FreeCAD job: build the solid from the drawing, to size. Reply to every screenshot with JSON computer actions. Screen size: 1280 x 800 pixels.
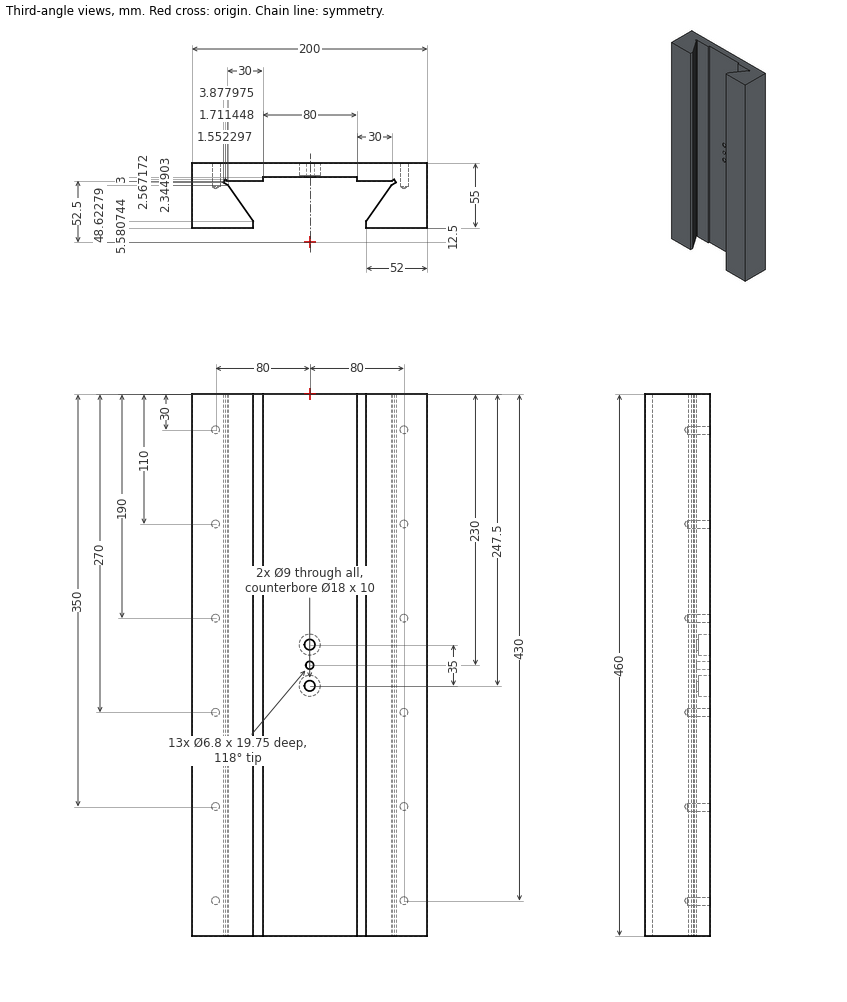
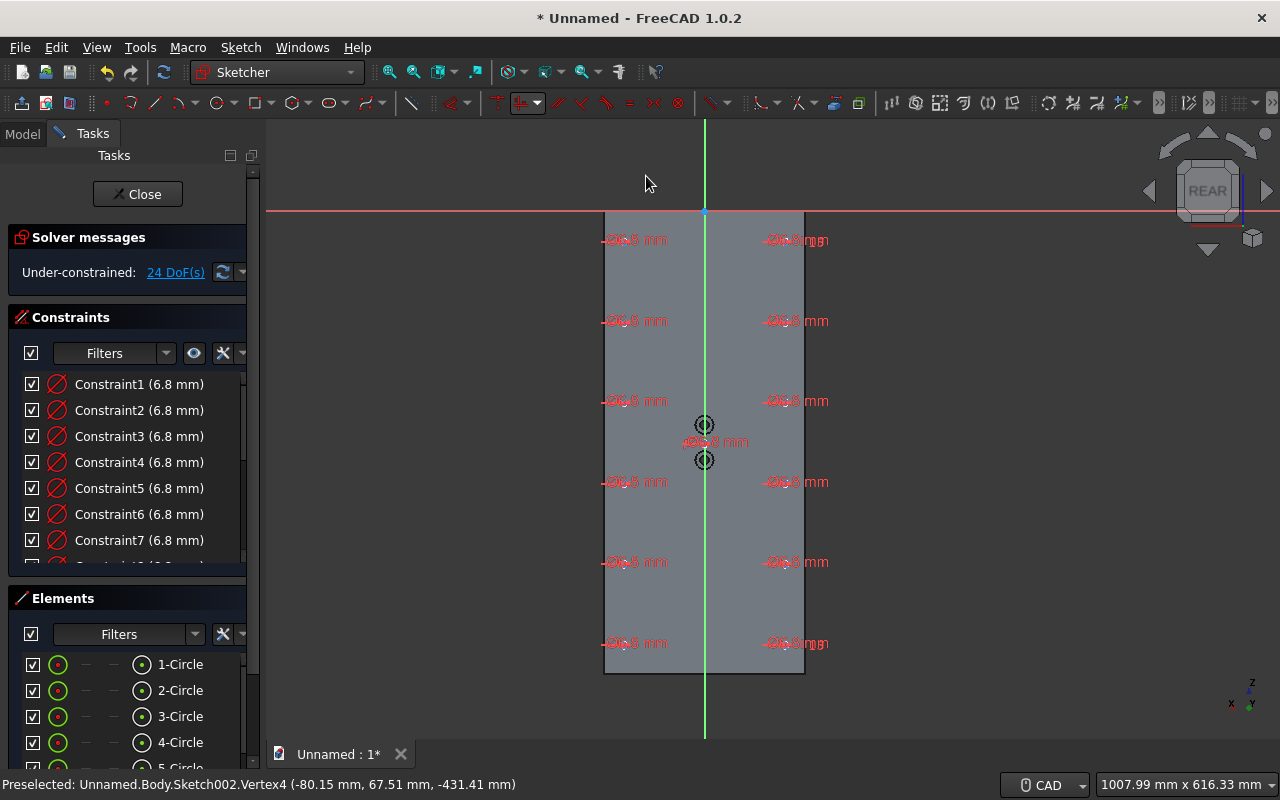
{"action": "left_click", "coordinate": [624, 645]}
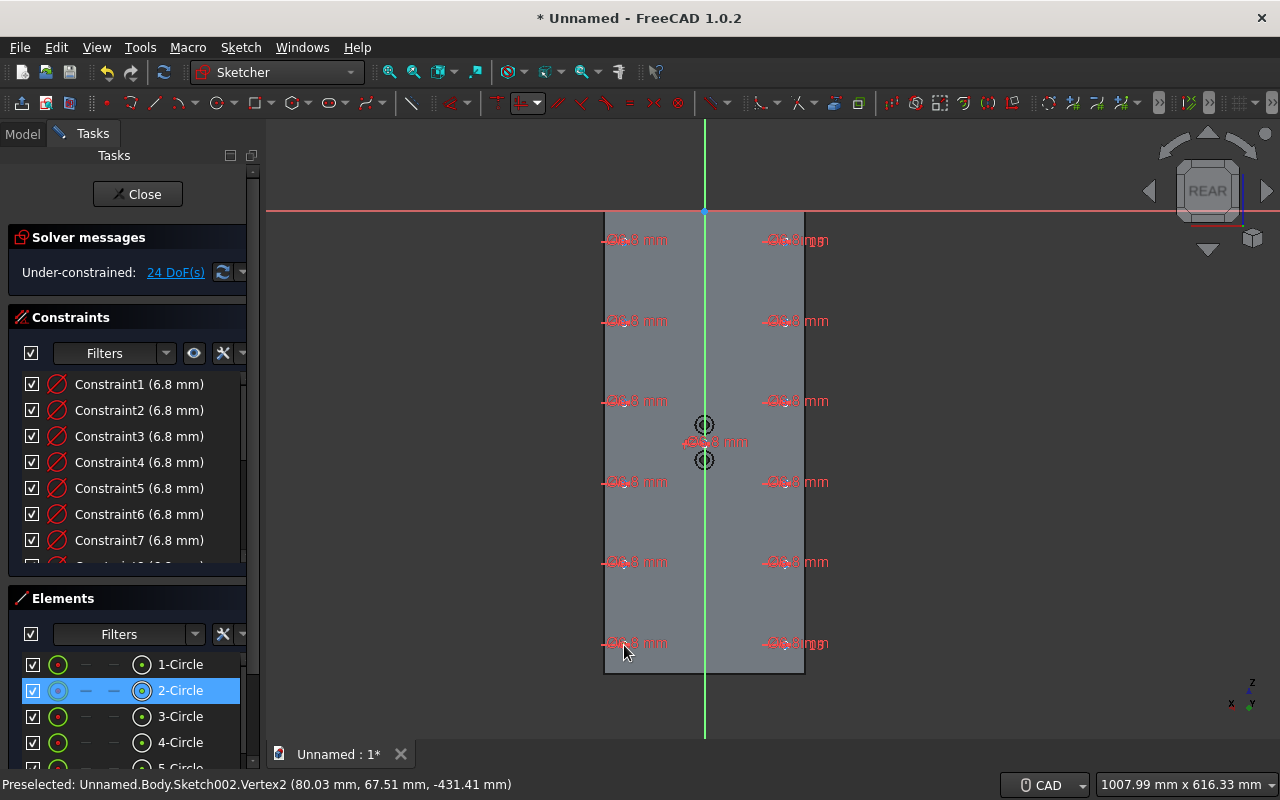
{"action": "left_click", "coordinate": [785, 645]}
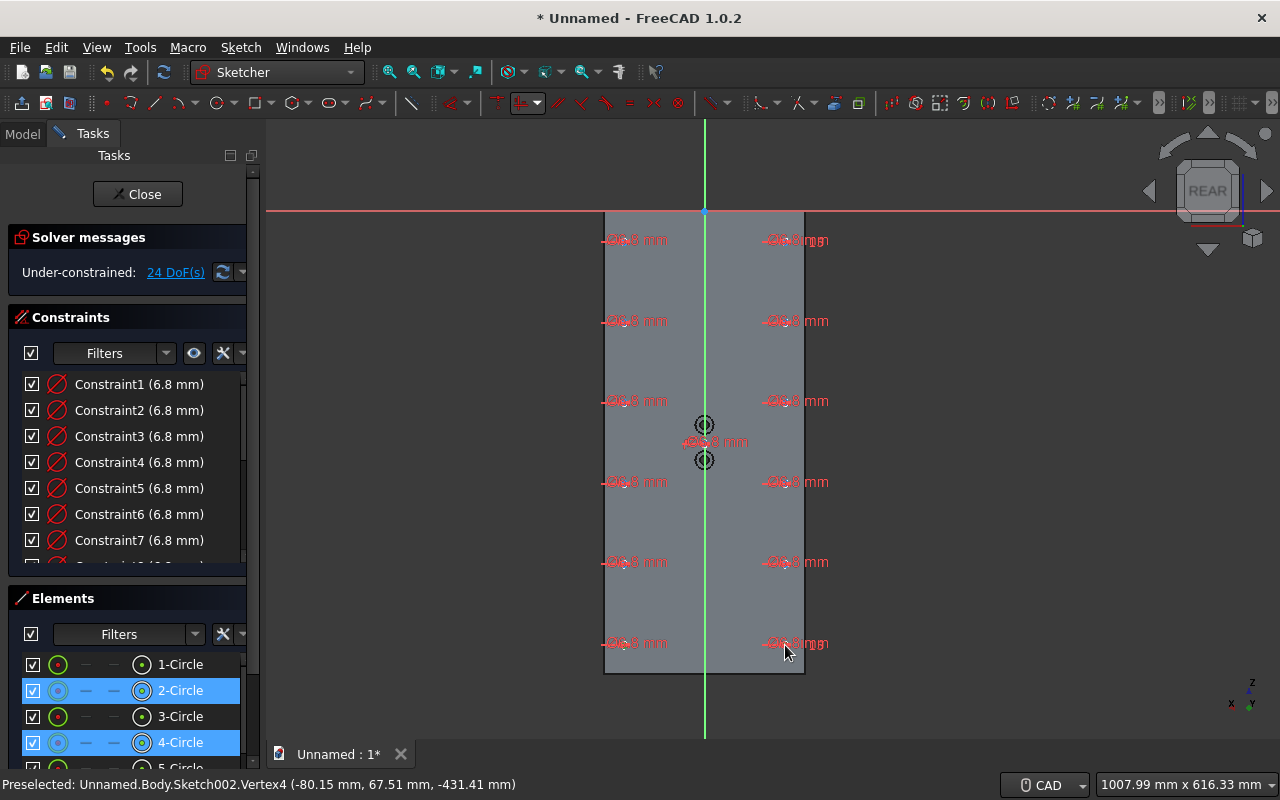
{"action": "key", "text": "h"}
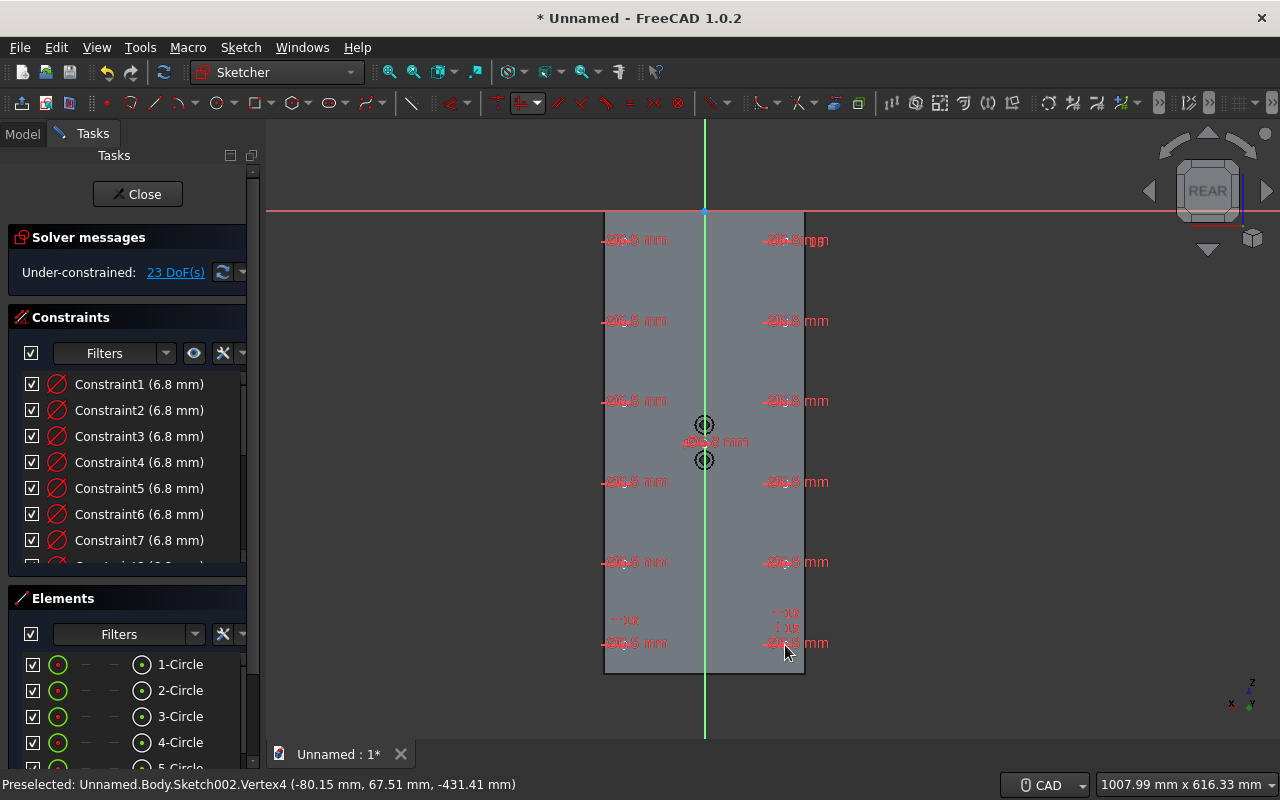
{"action": "left_click", "coordinate": [624, 645]}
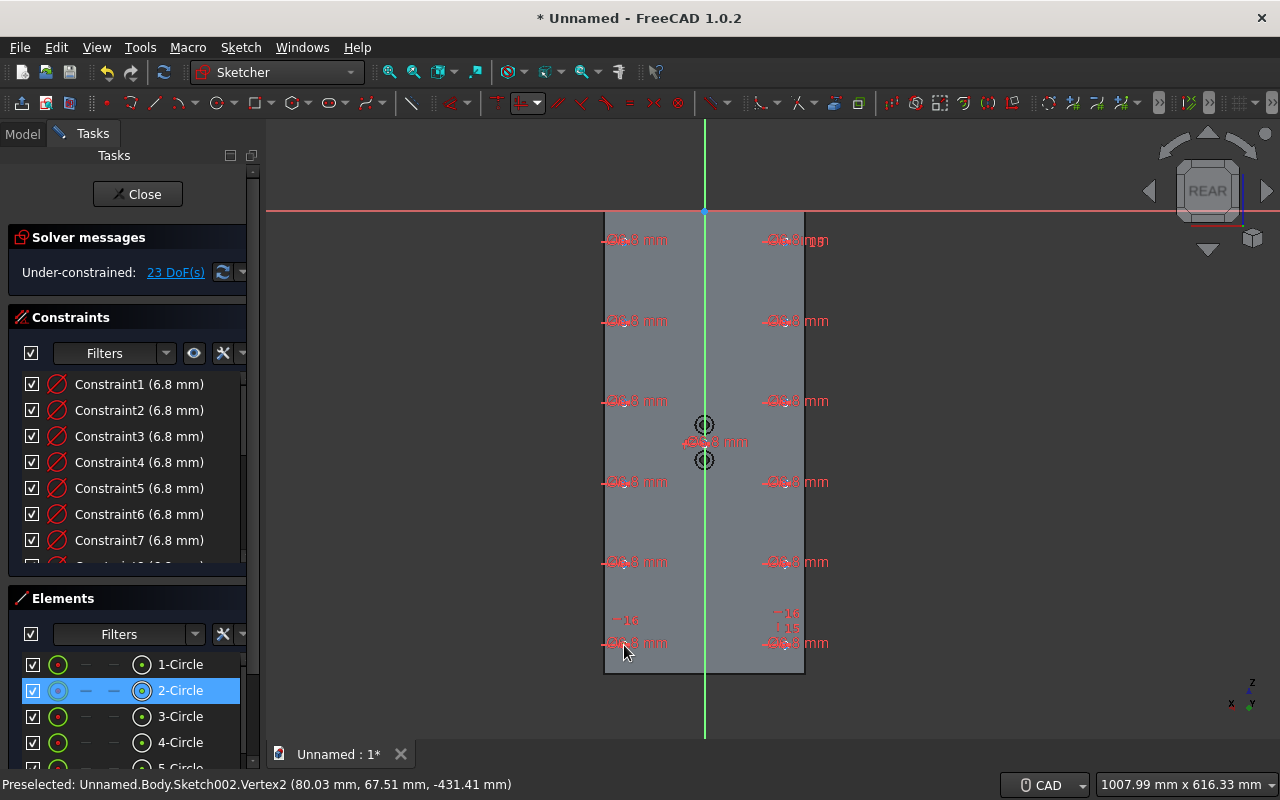
{"action": "left_click", "coordinate": [624, 242]}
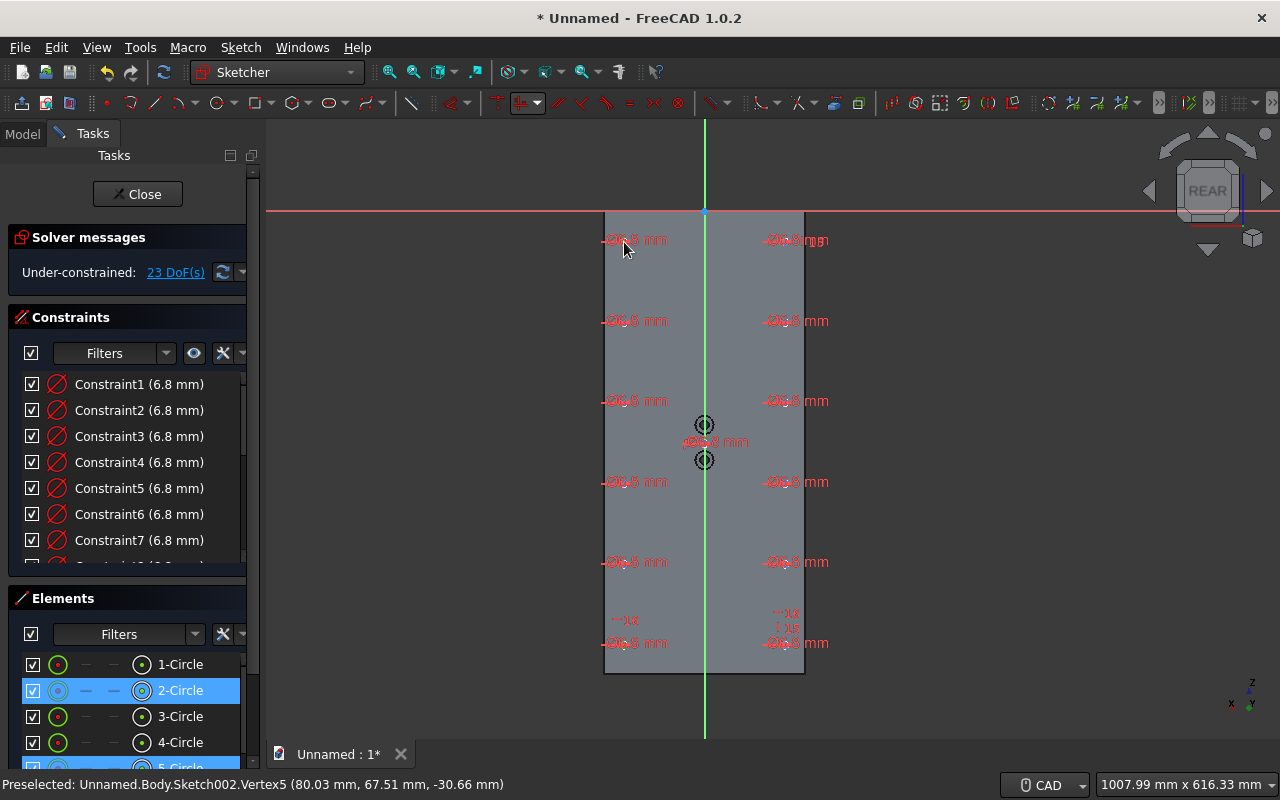
{"action": "key", "text": "v"}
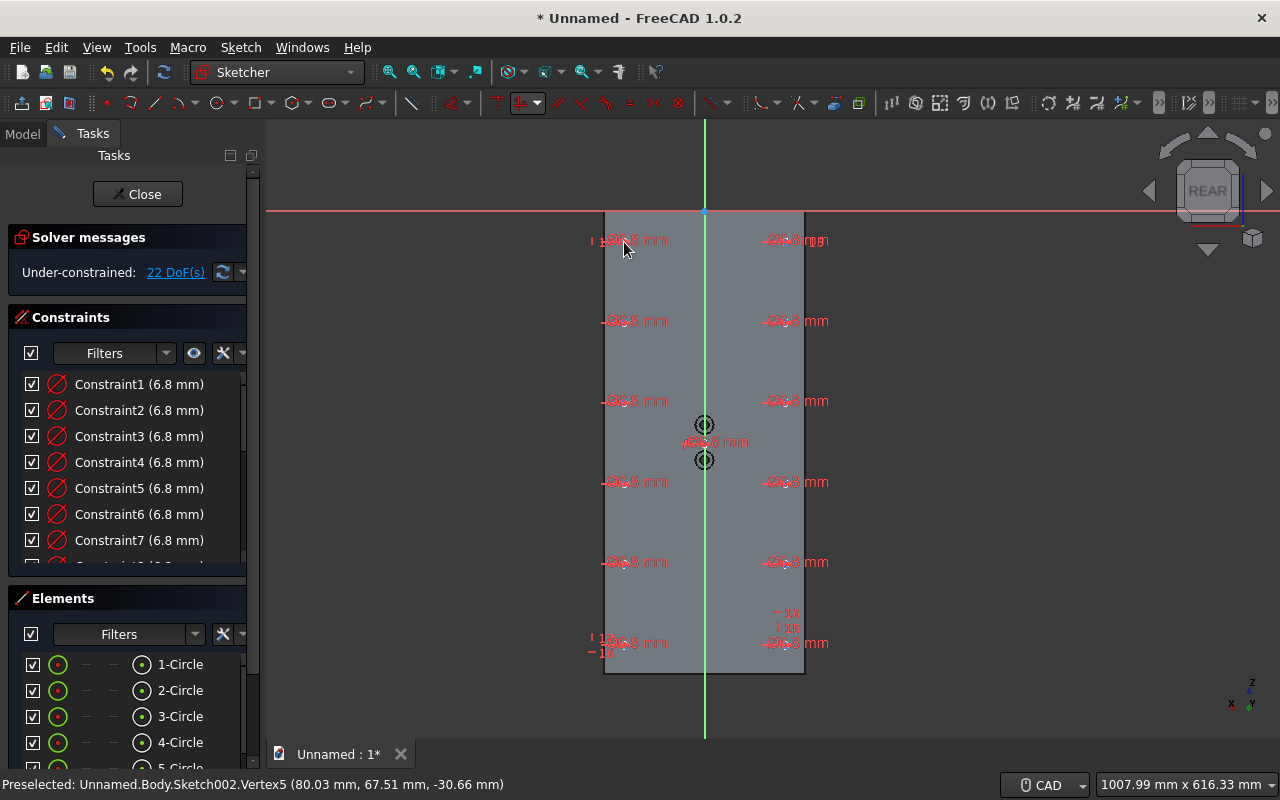
{"action": "left_click", "coordinate": [785, 242]}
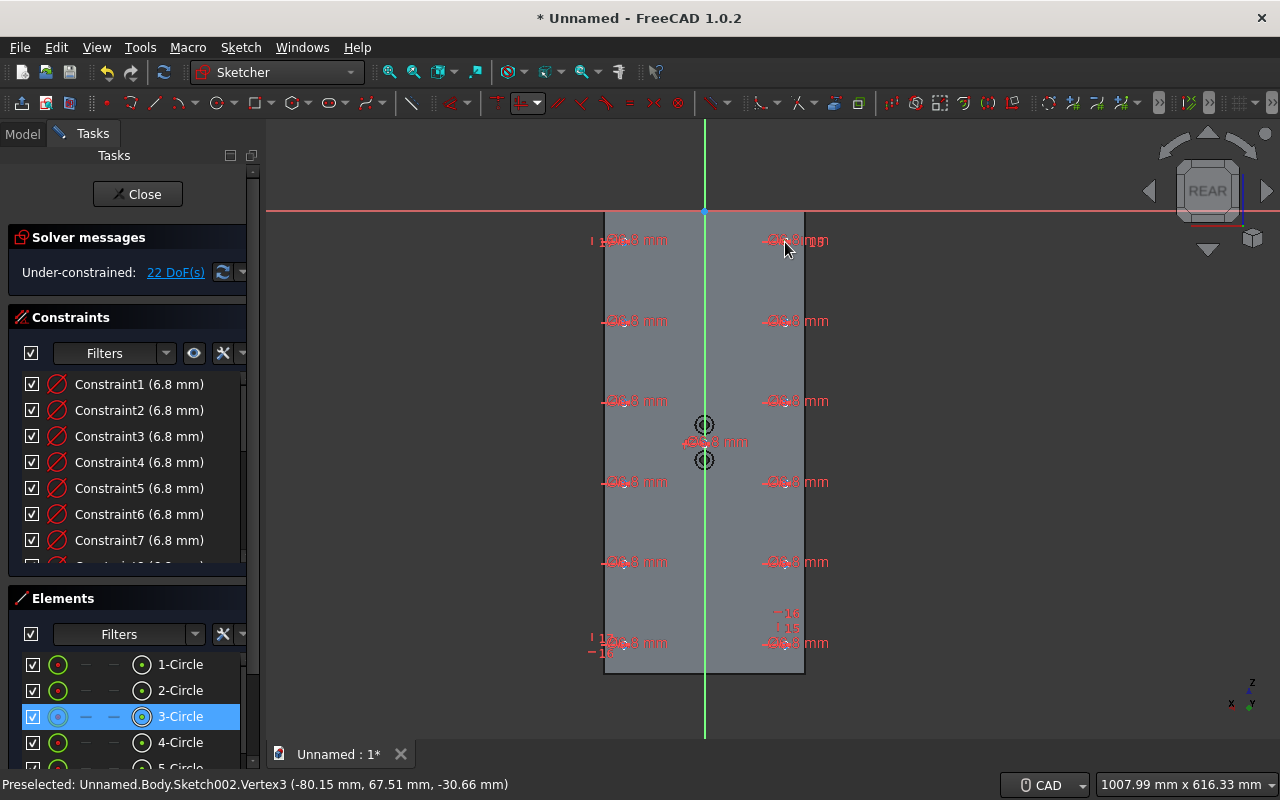
{"action": "left_click", "coordinate": [624, 242]}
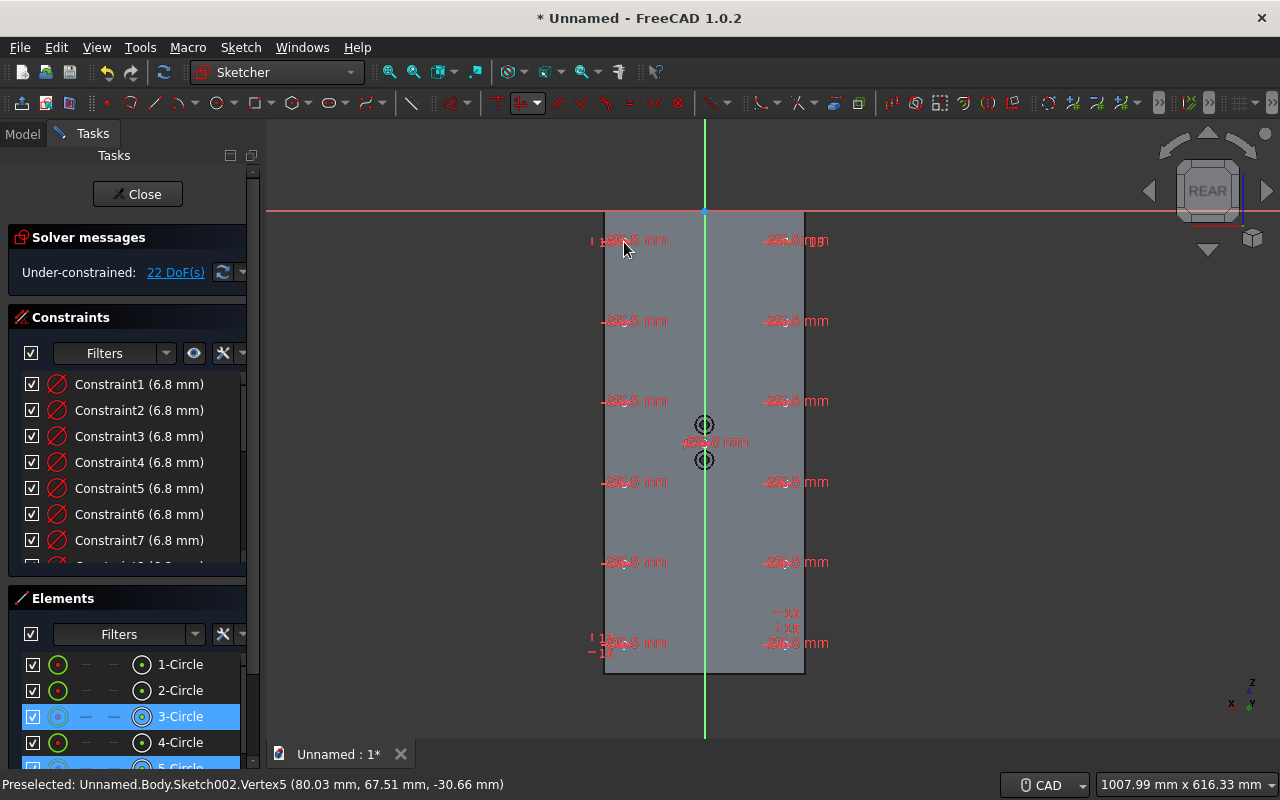
{"action": "left_click", "coordinate": [540, 104]}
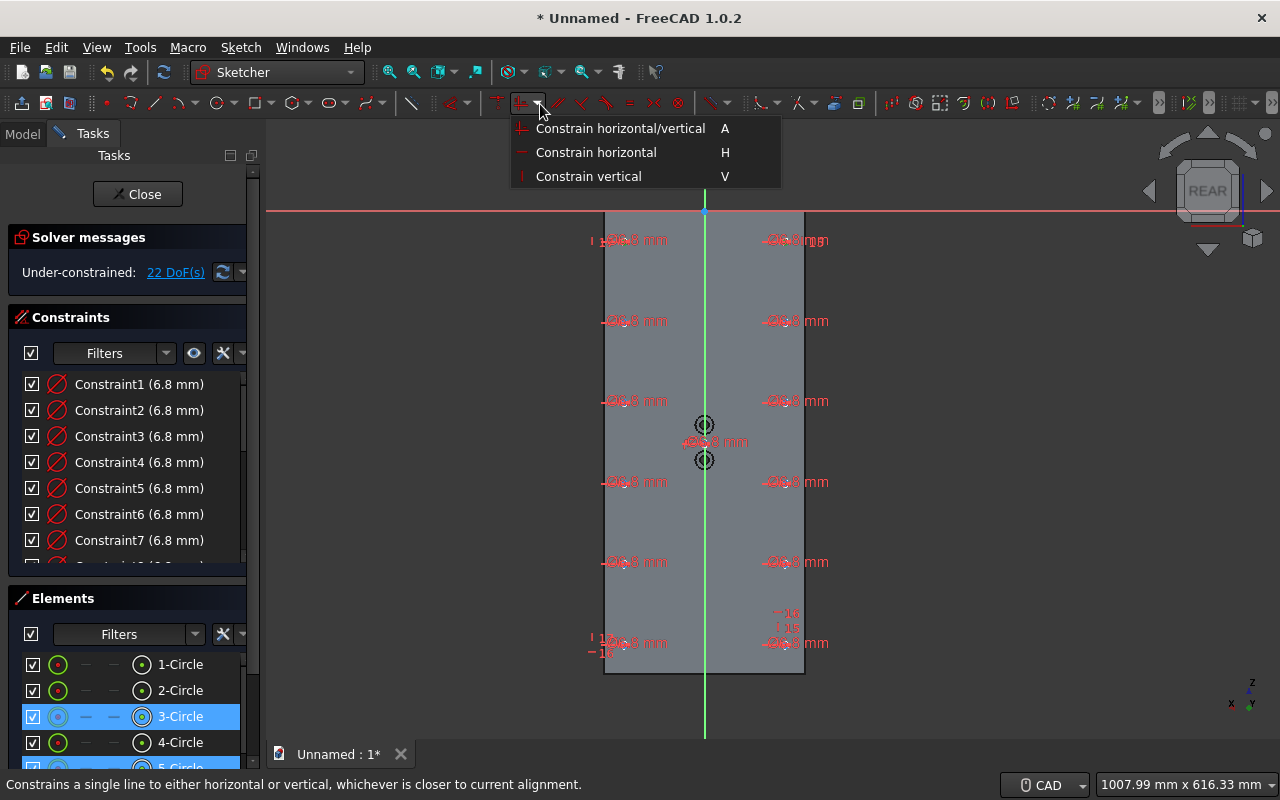
{"action": "left_click", "coordinate": [646, 152]}